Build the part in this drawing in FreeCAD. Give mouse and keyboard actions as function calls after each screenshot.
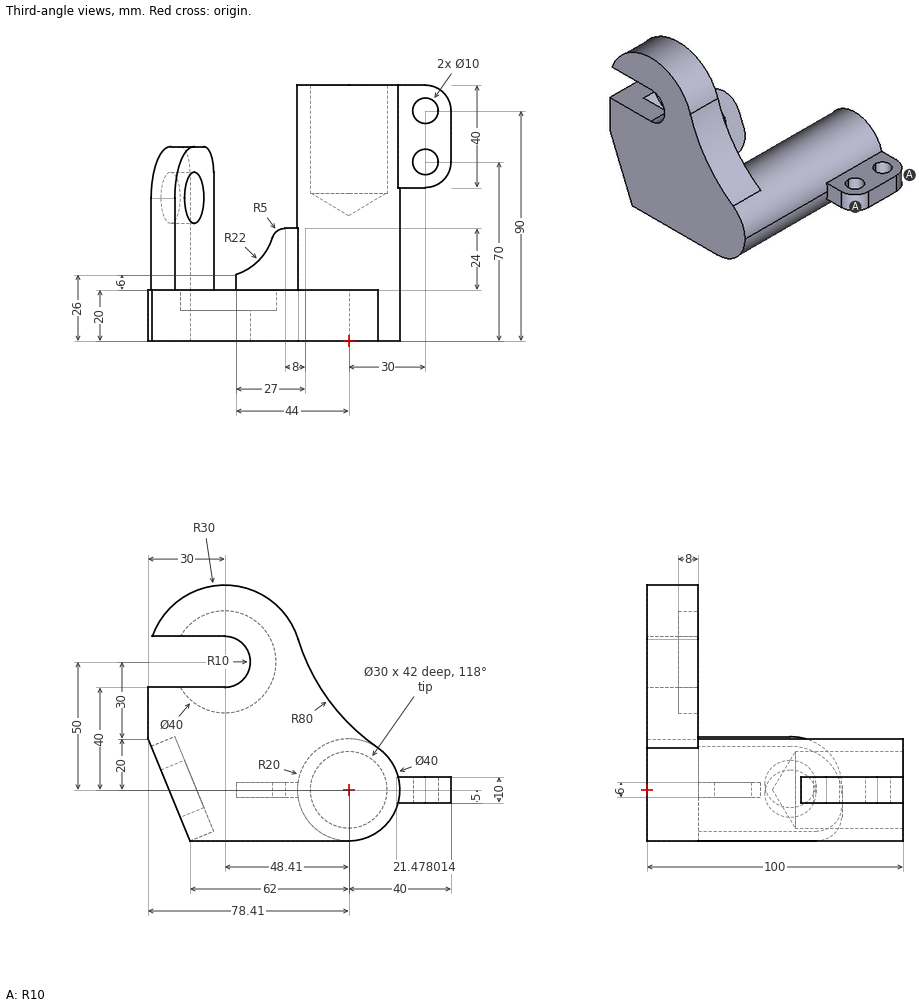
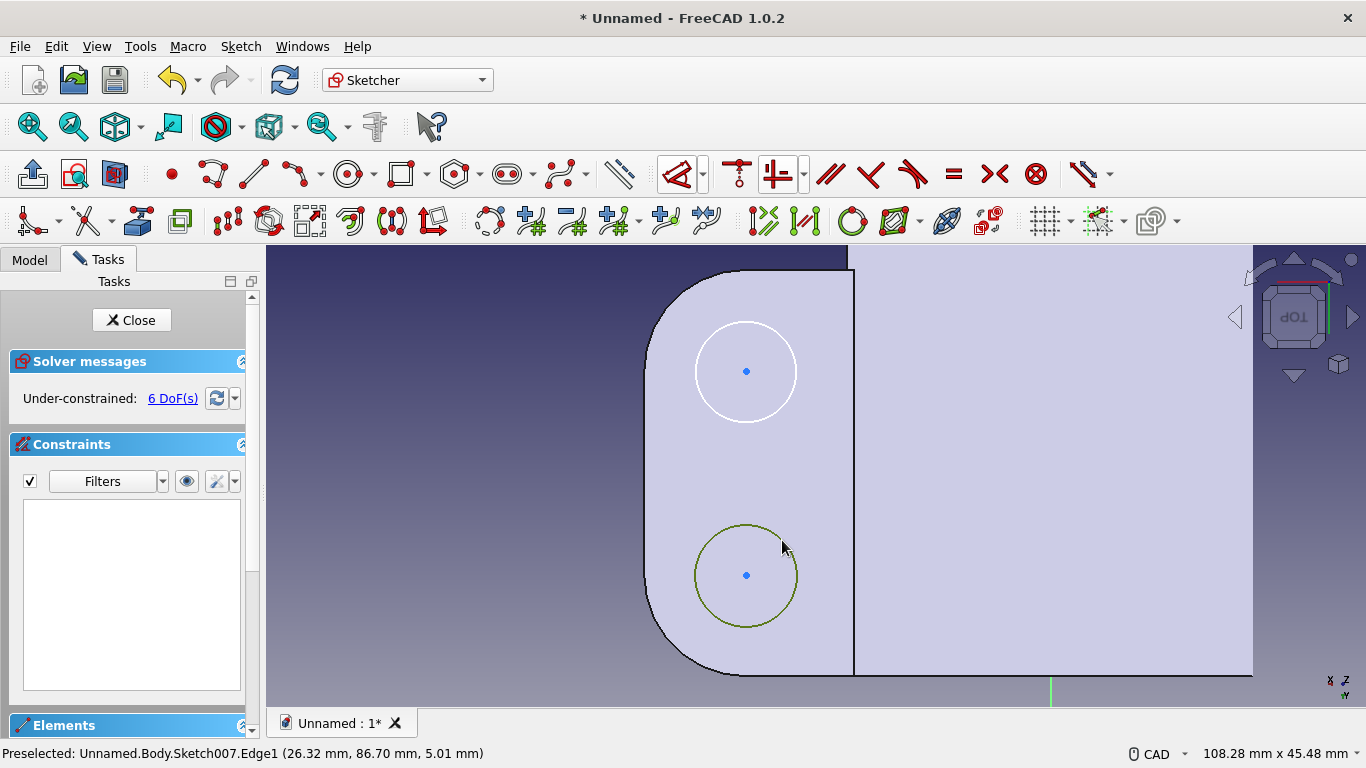
click(781, 336)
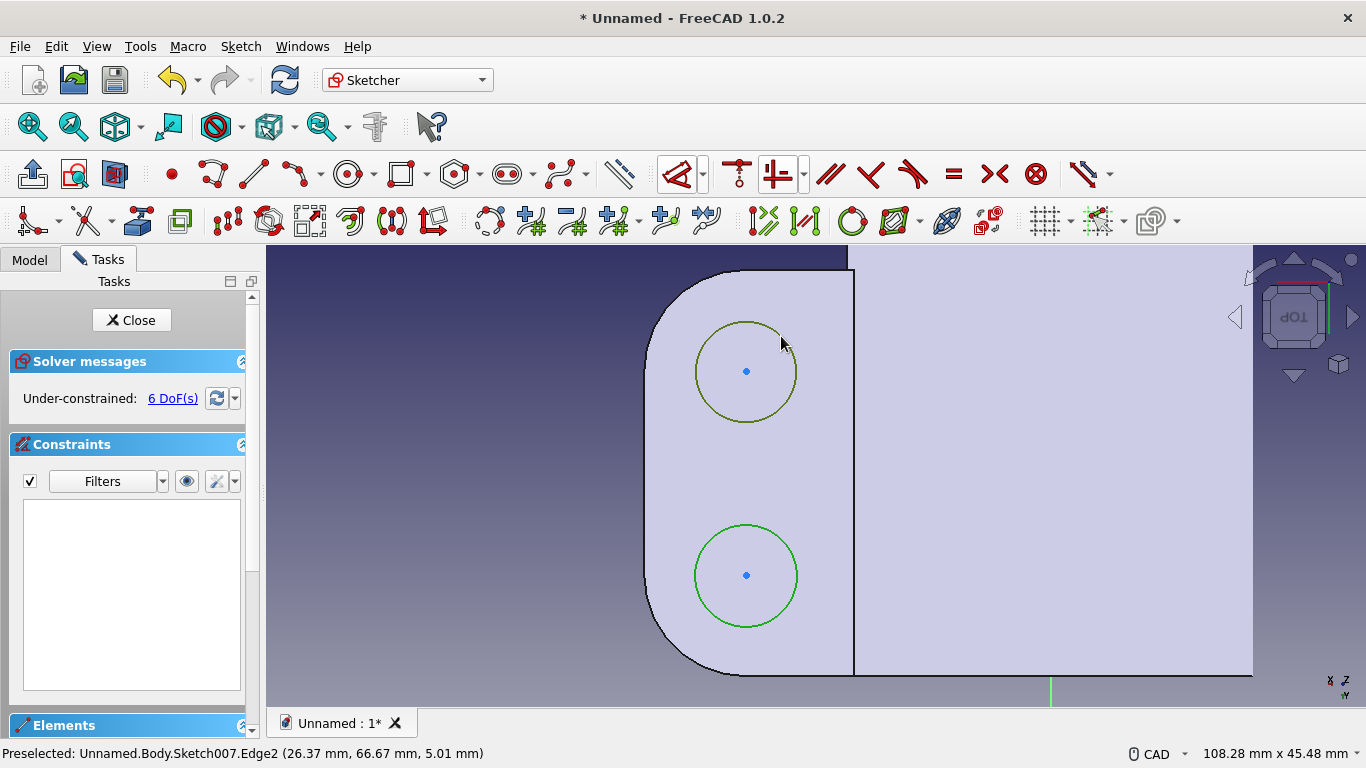
key(e)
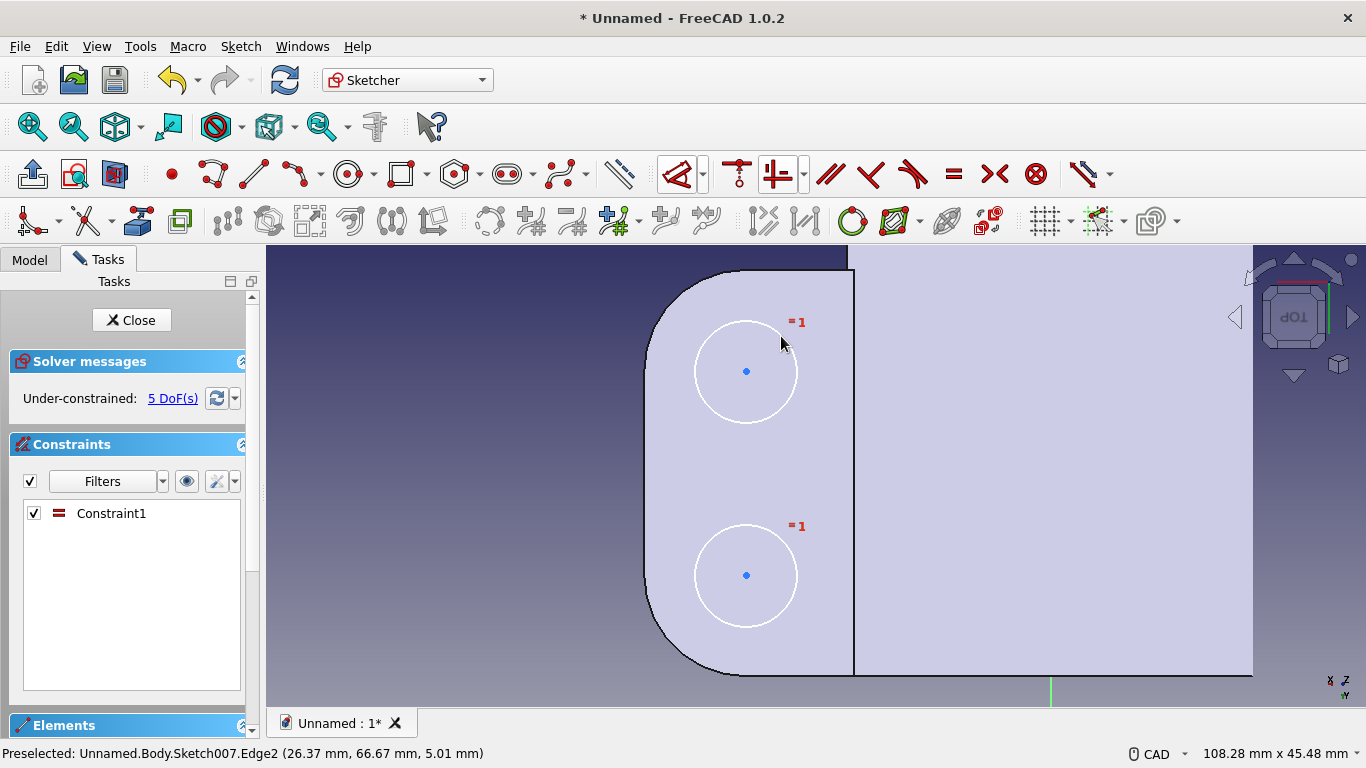
click(746, 576)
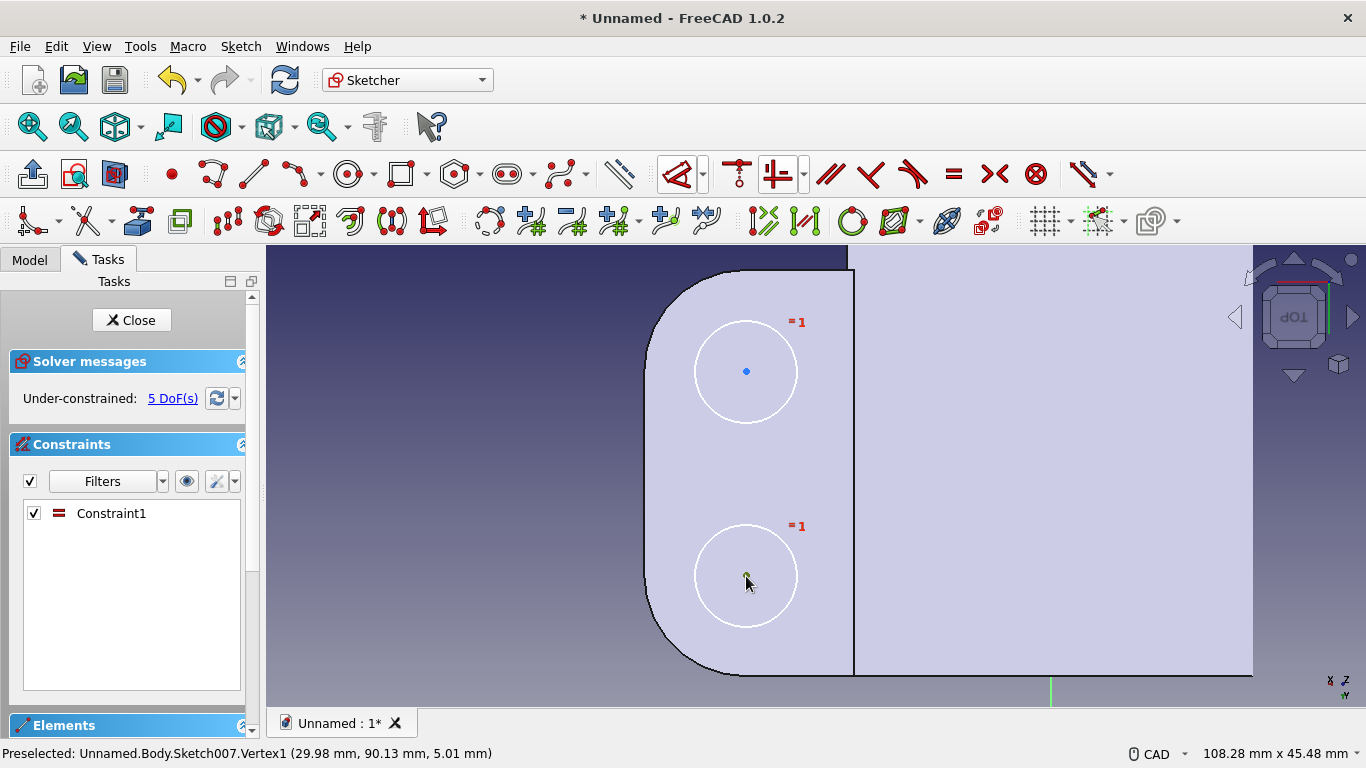
click(746, 372)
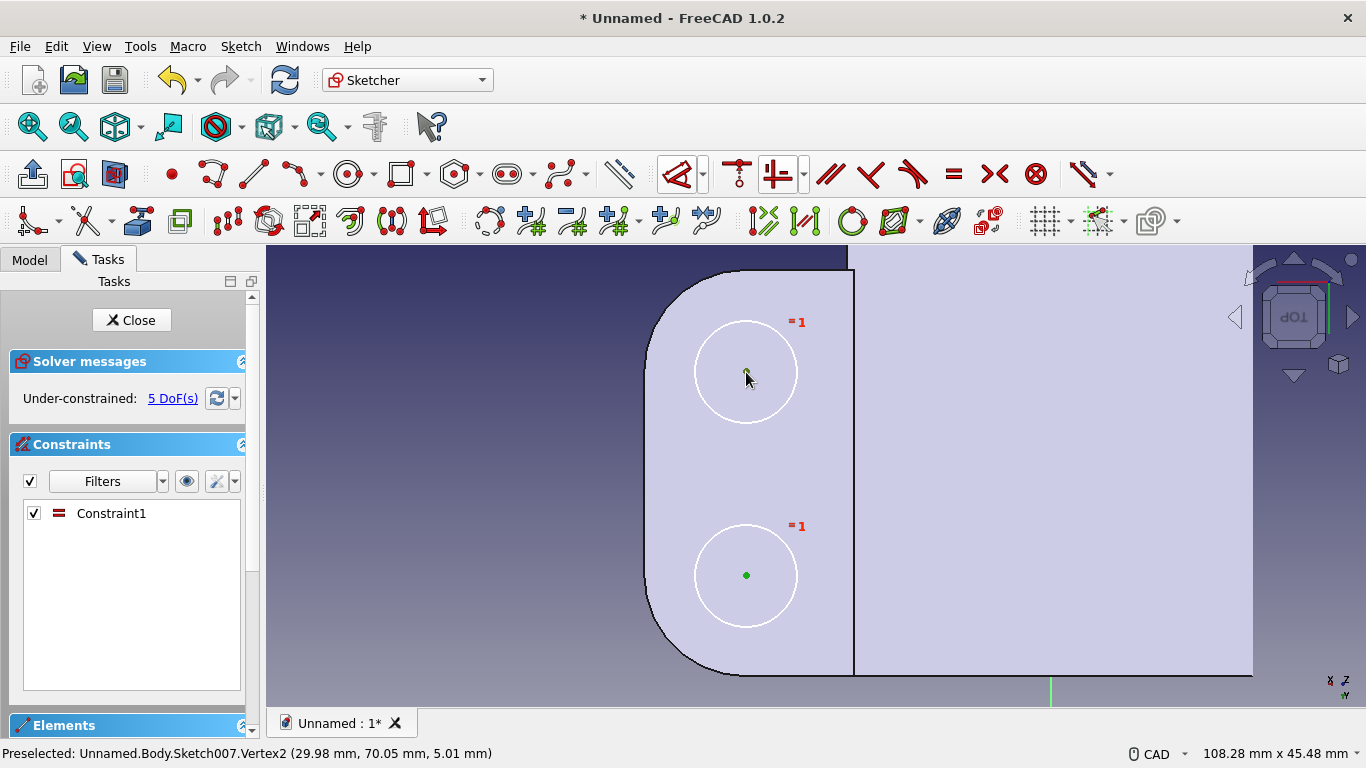
key(v)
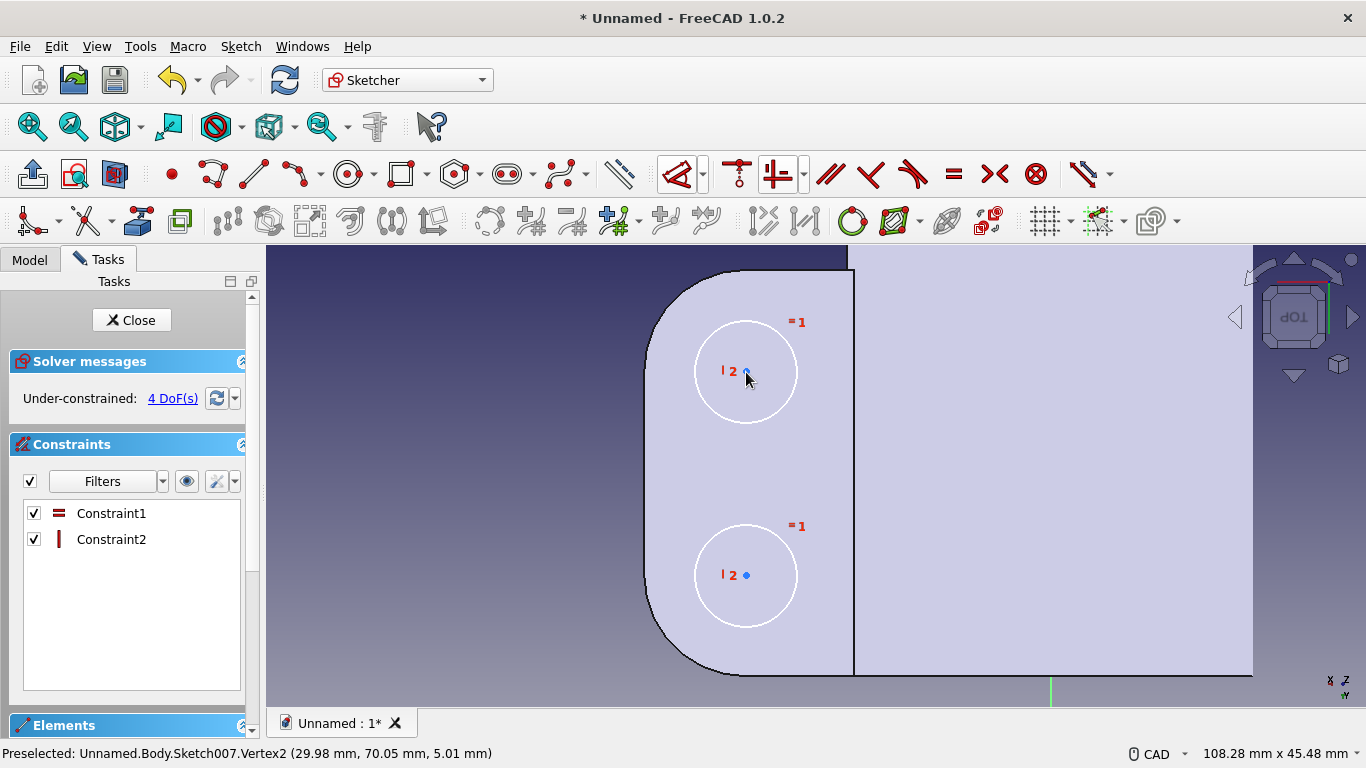
key(d)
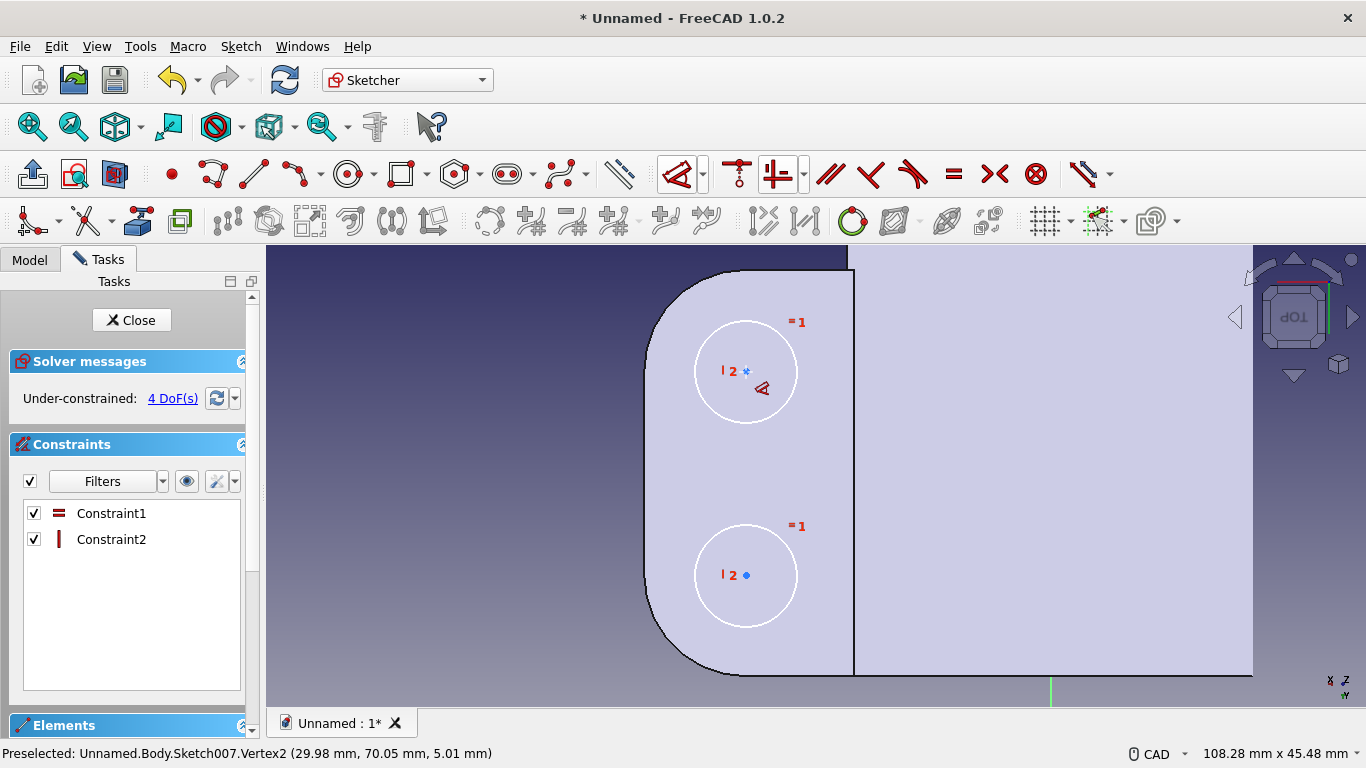
click(782, 540)
click(805, 517)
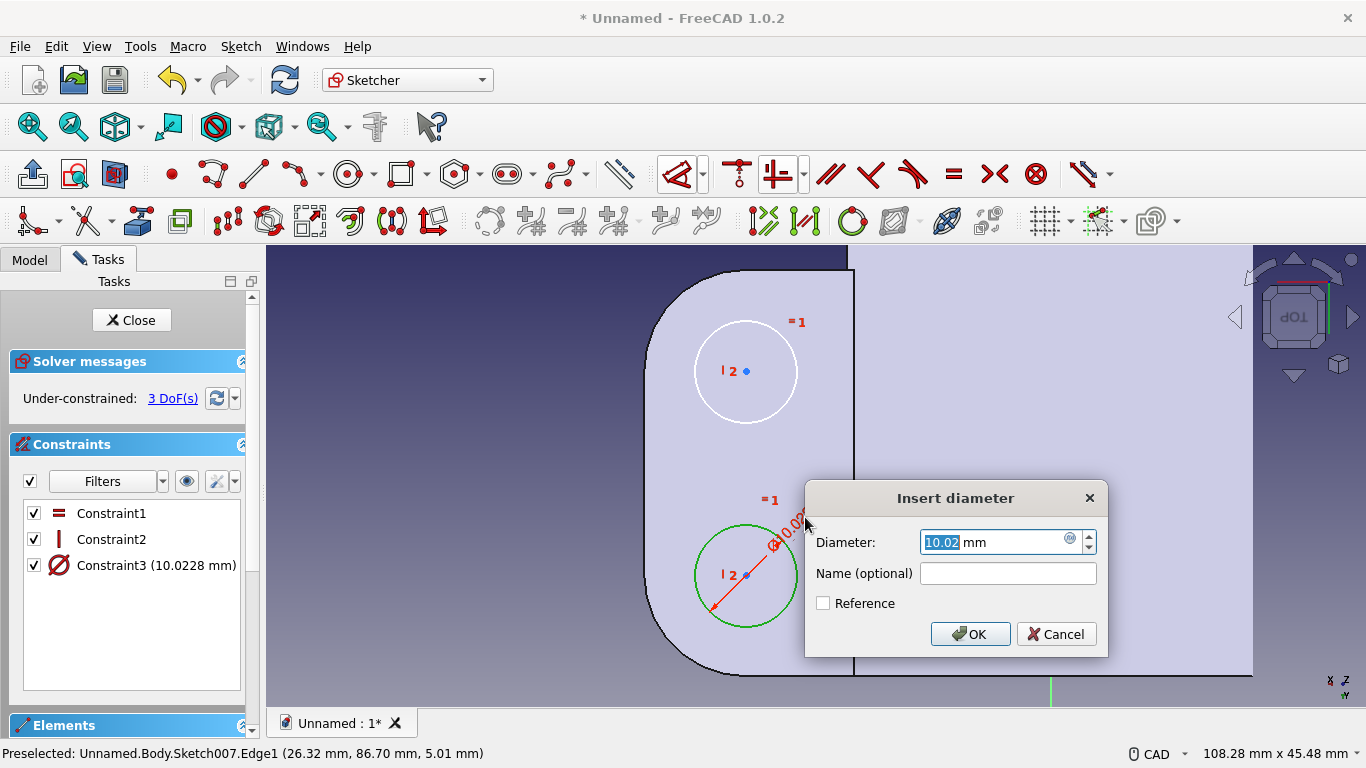
text(10)
key(Return)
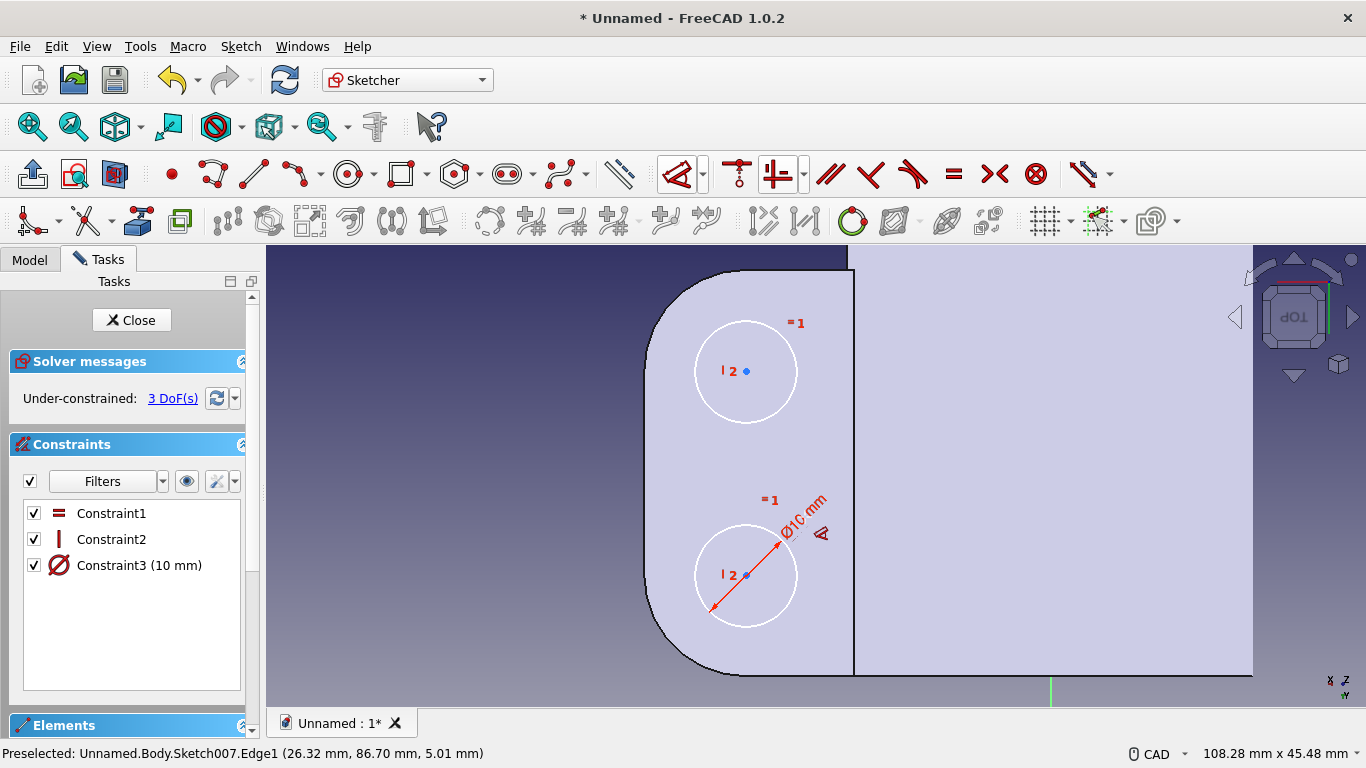
click(746, 576)
click(898, 610)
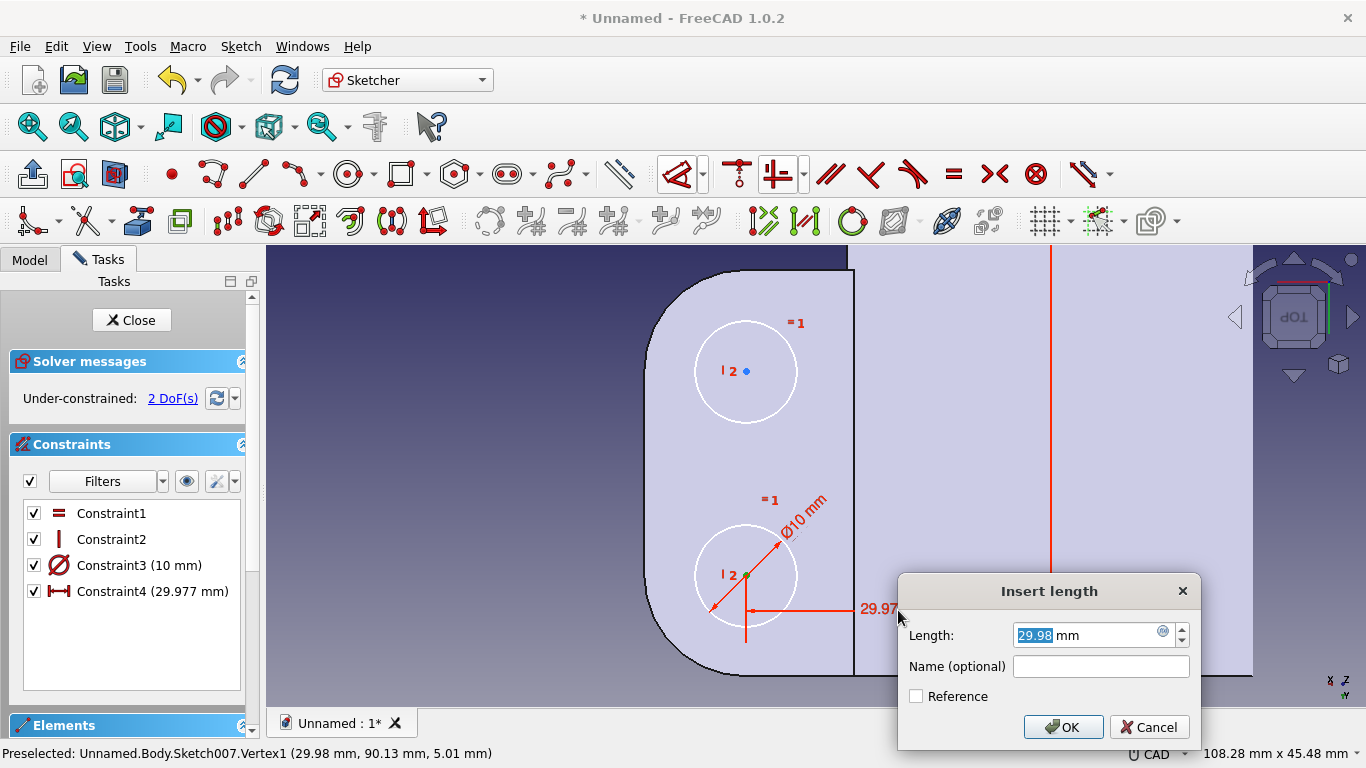
text(30)
key(Return)